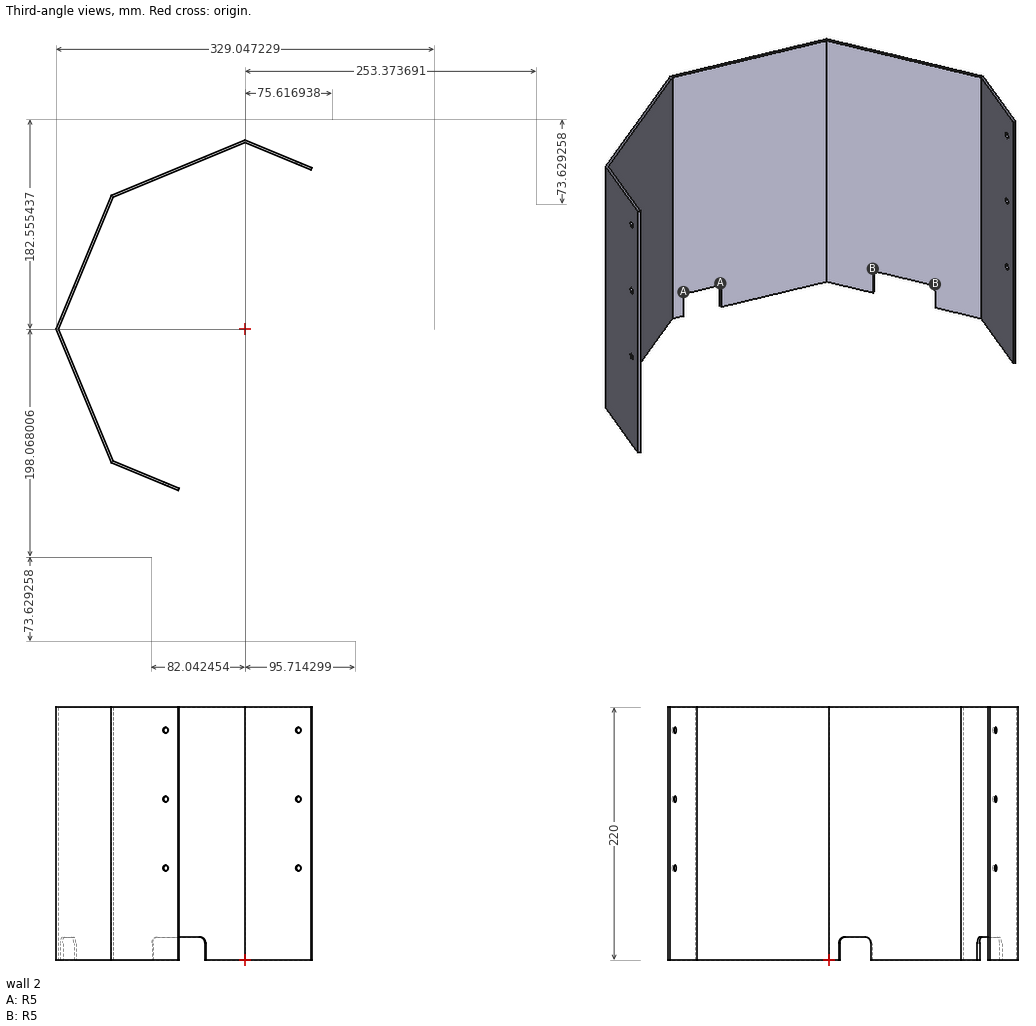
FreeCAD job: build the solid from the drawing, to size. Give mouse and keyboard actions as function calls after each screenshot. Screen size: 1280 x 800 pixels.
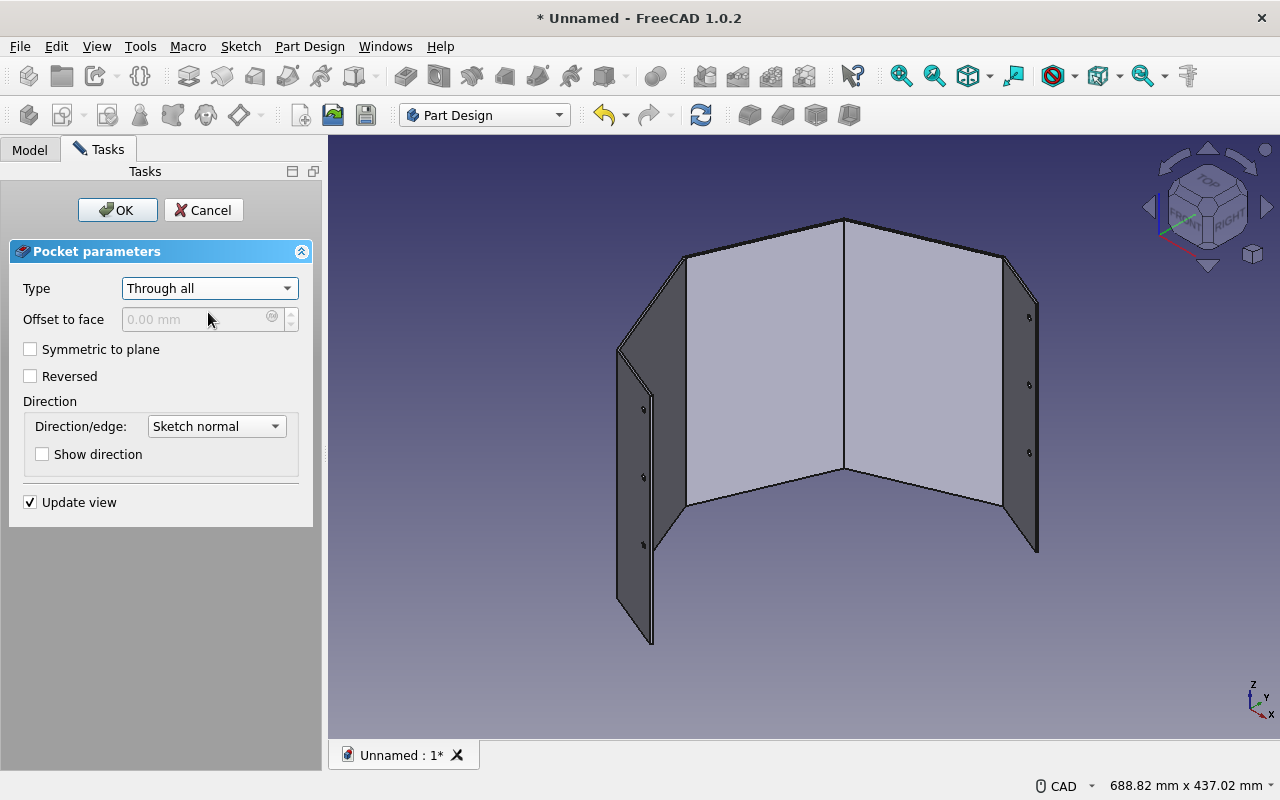
click(118, 210)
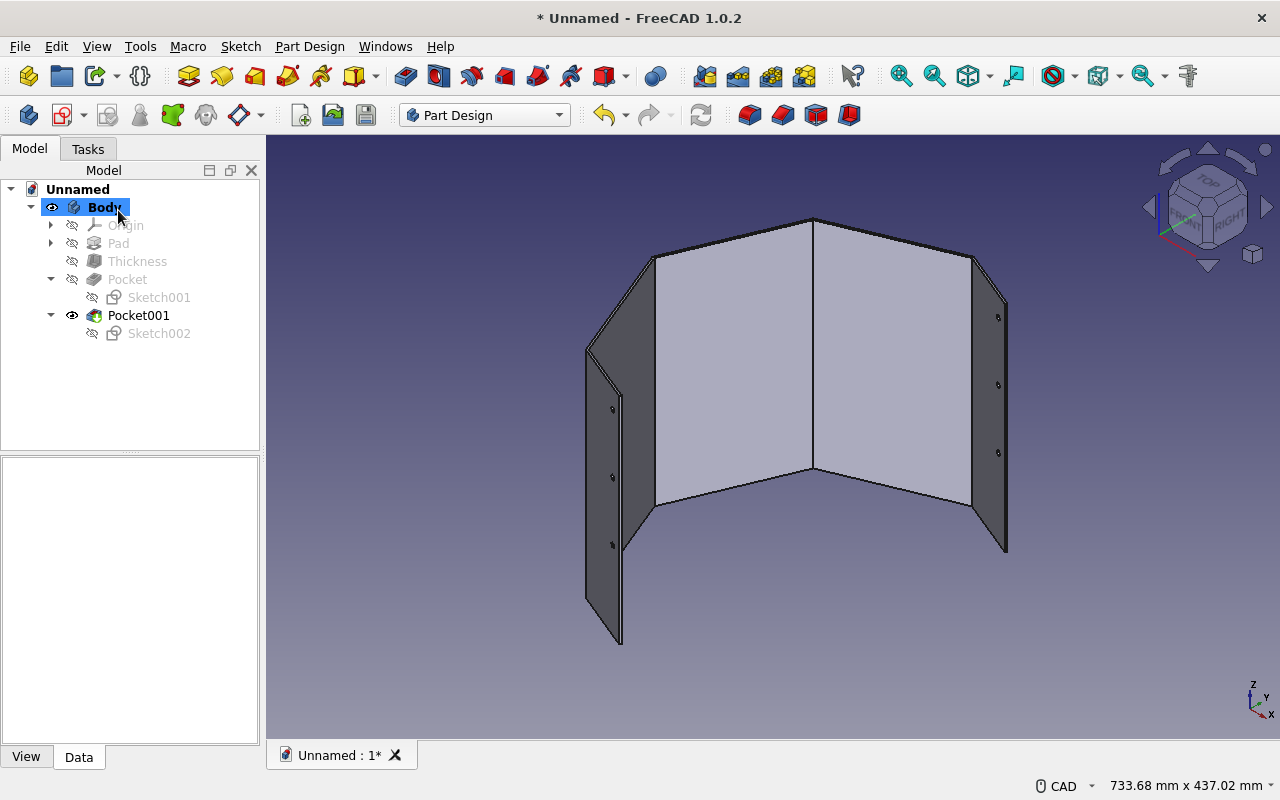
key(6)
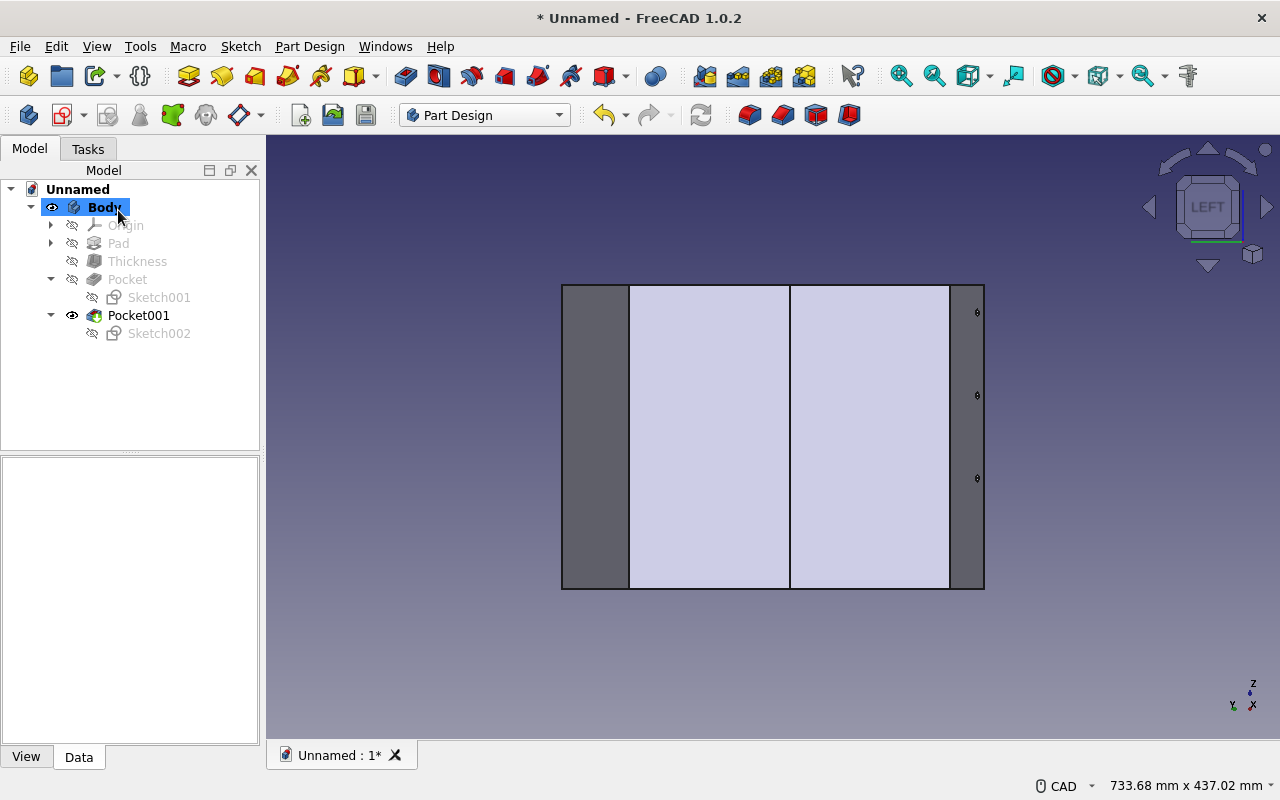
click(709, 393)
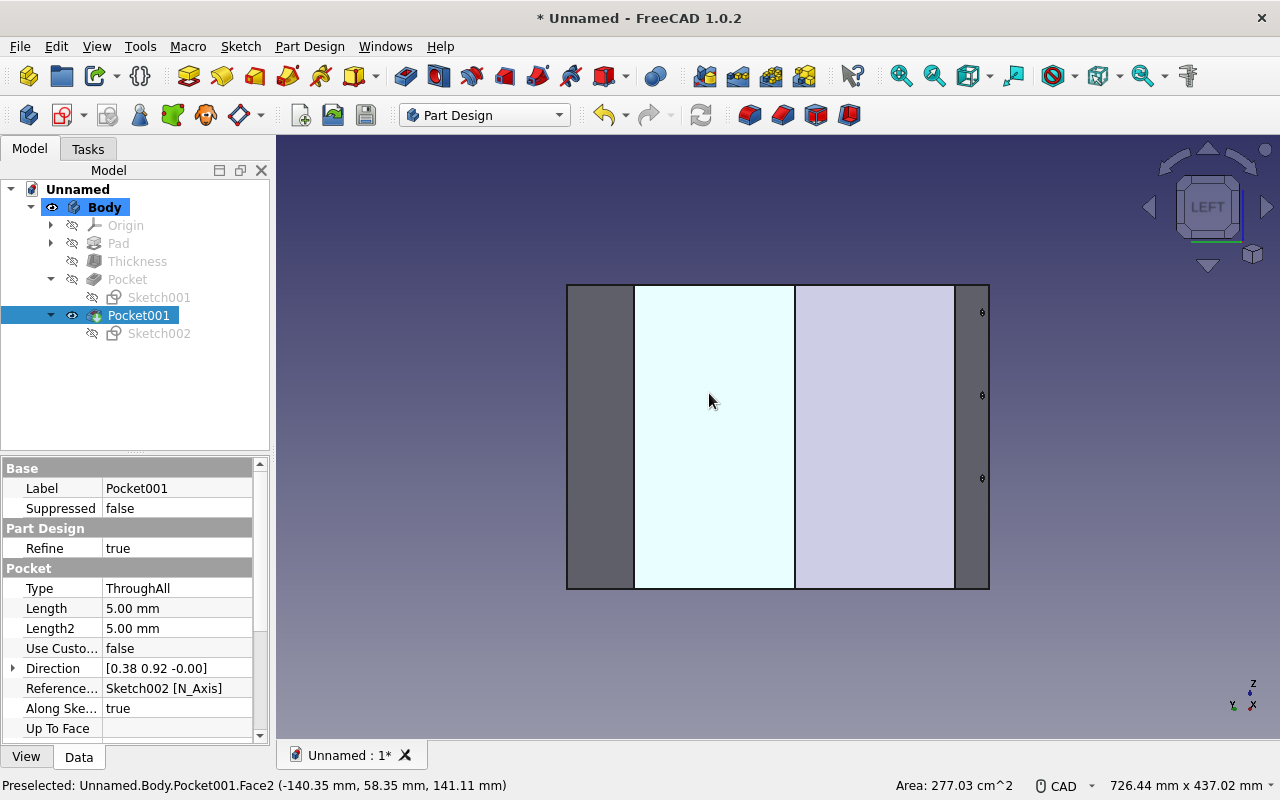
click(62, 116)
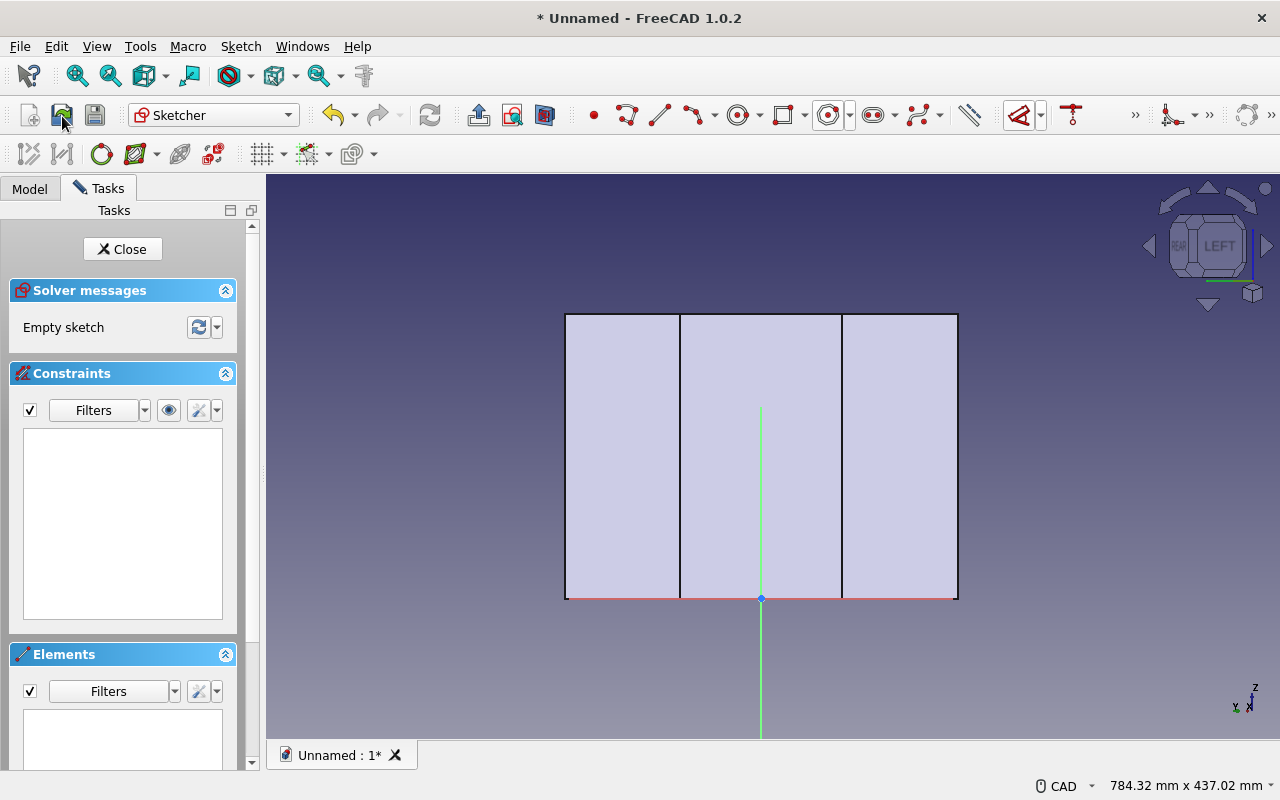
scroll(807, 602, up, 11)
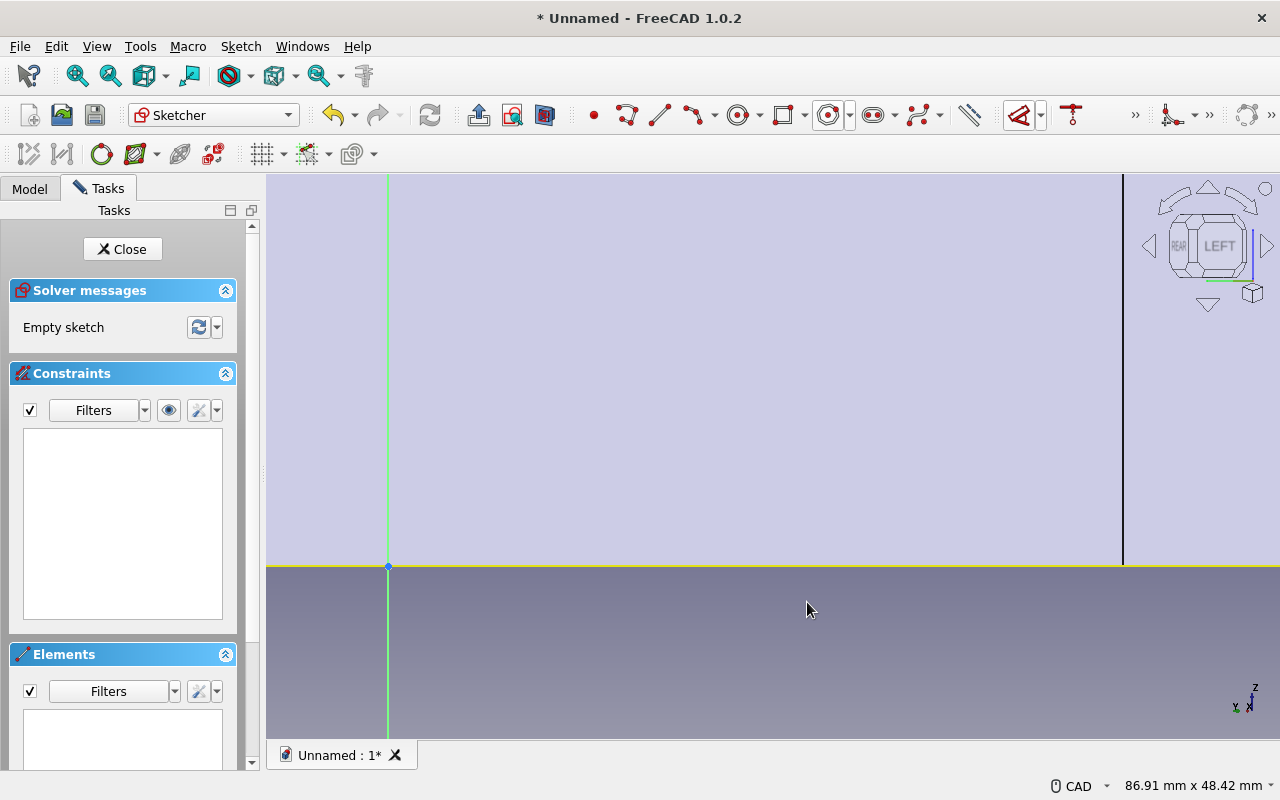
click(782, 116)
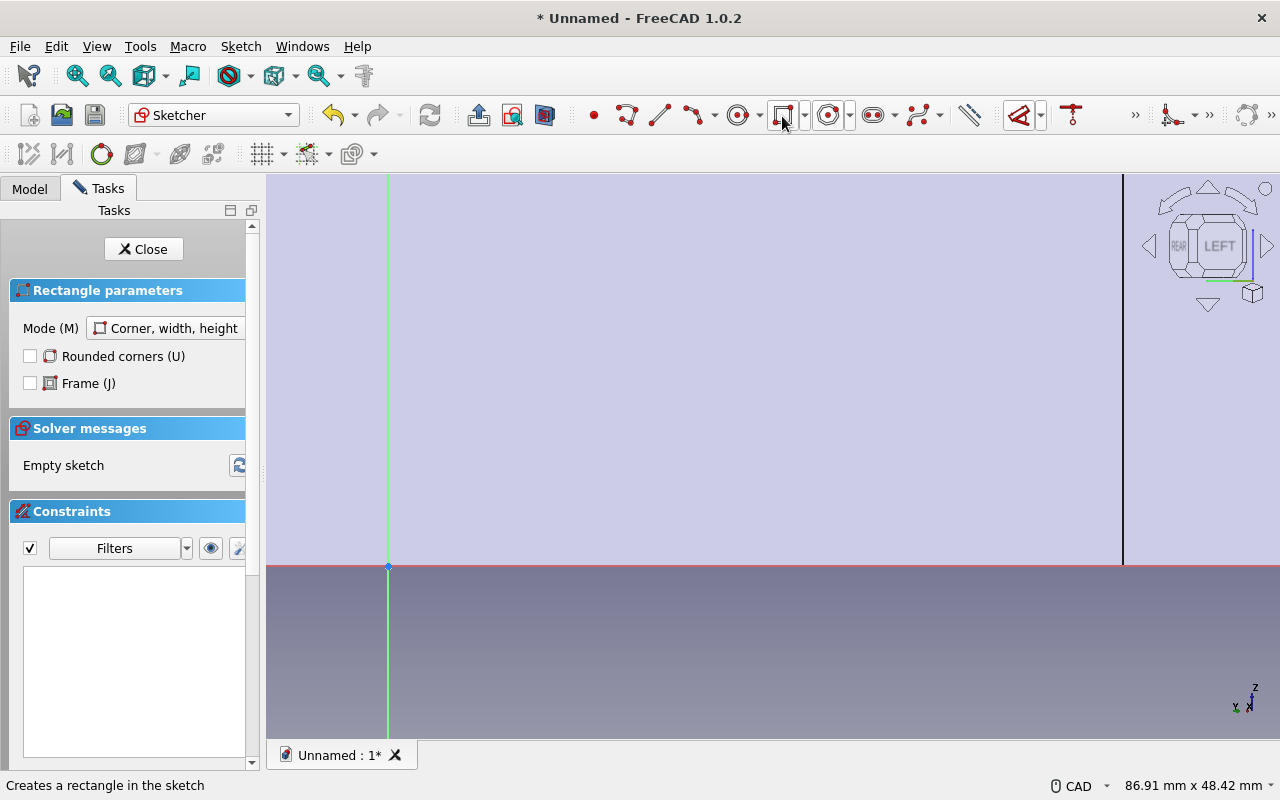
click(656, 333)
click(1006, 566)
key(Escape)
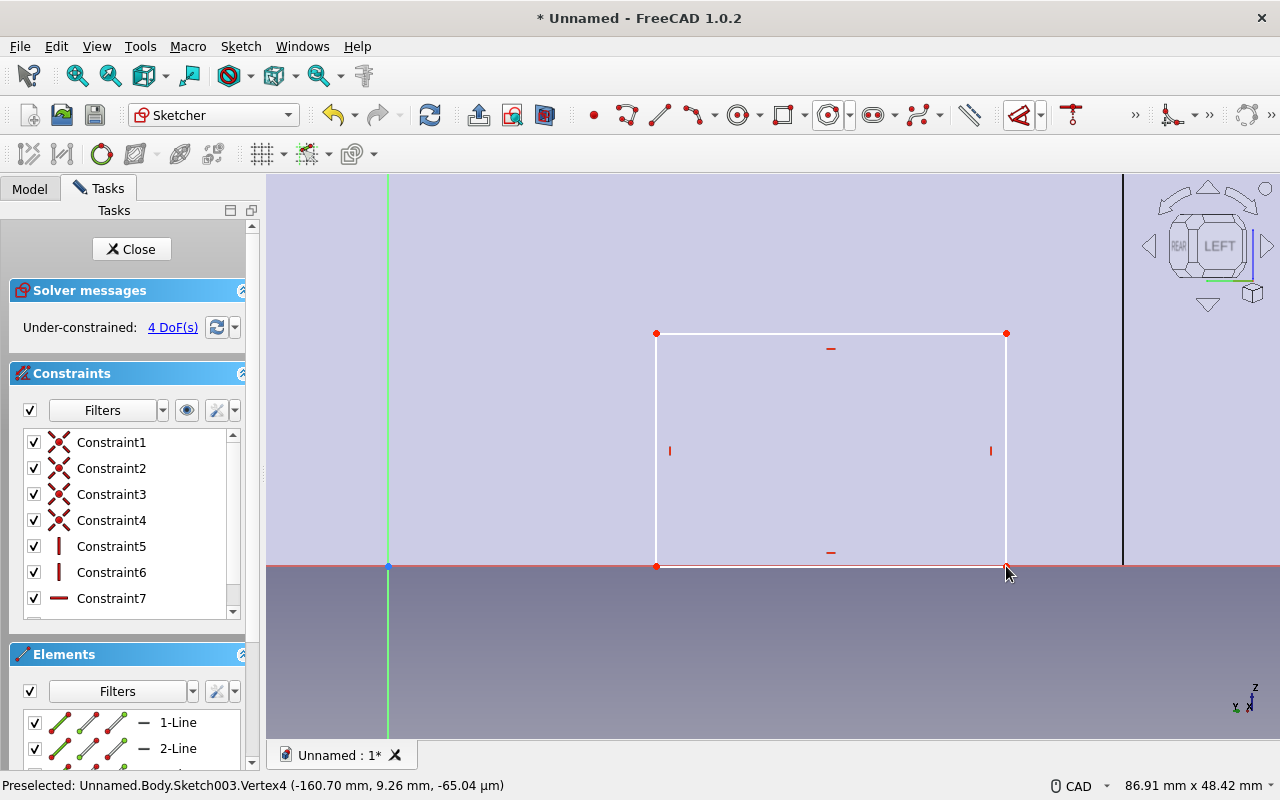
click(656, 567)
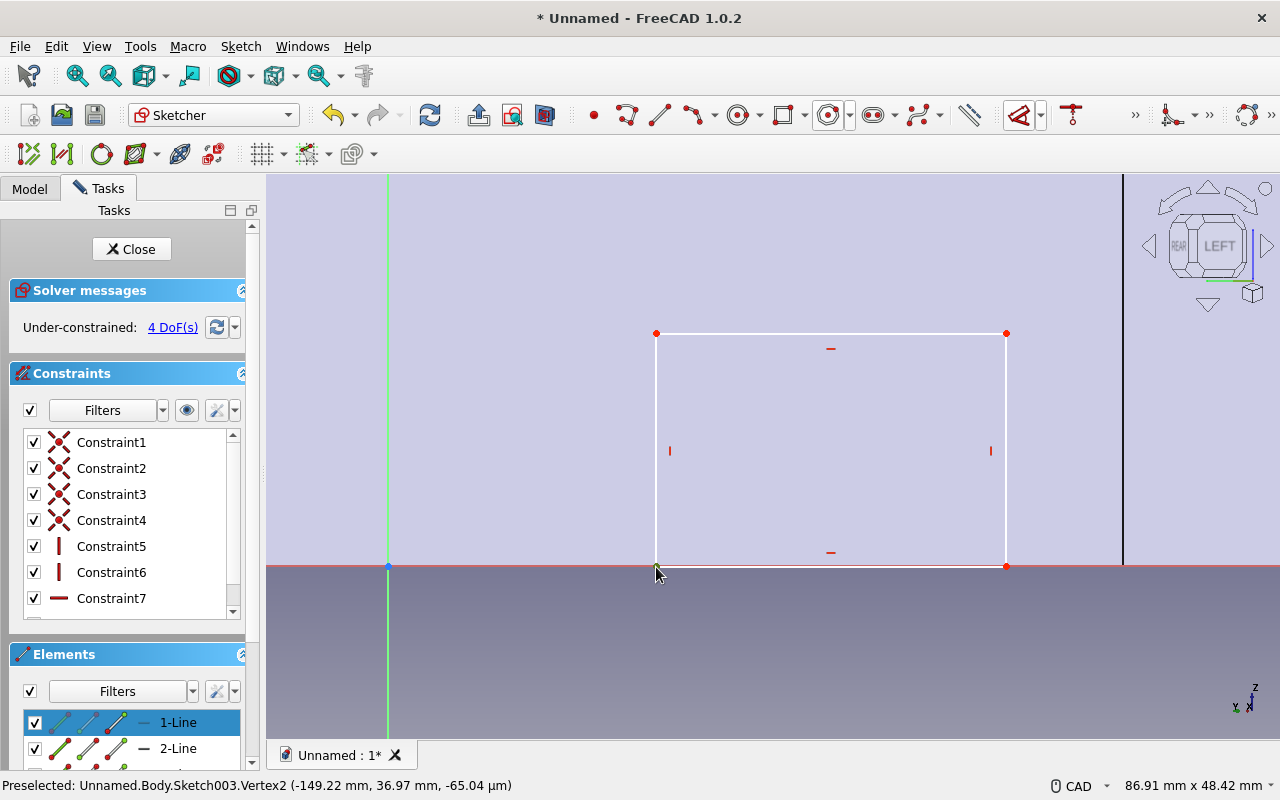
click(353, 566)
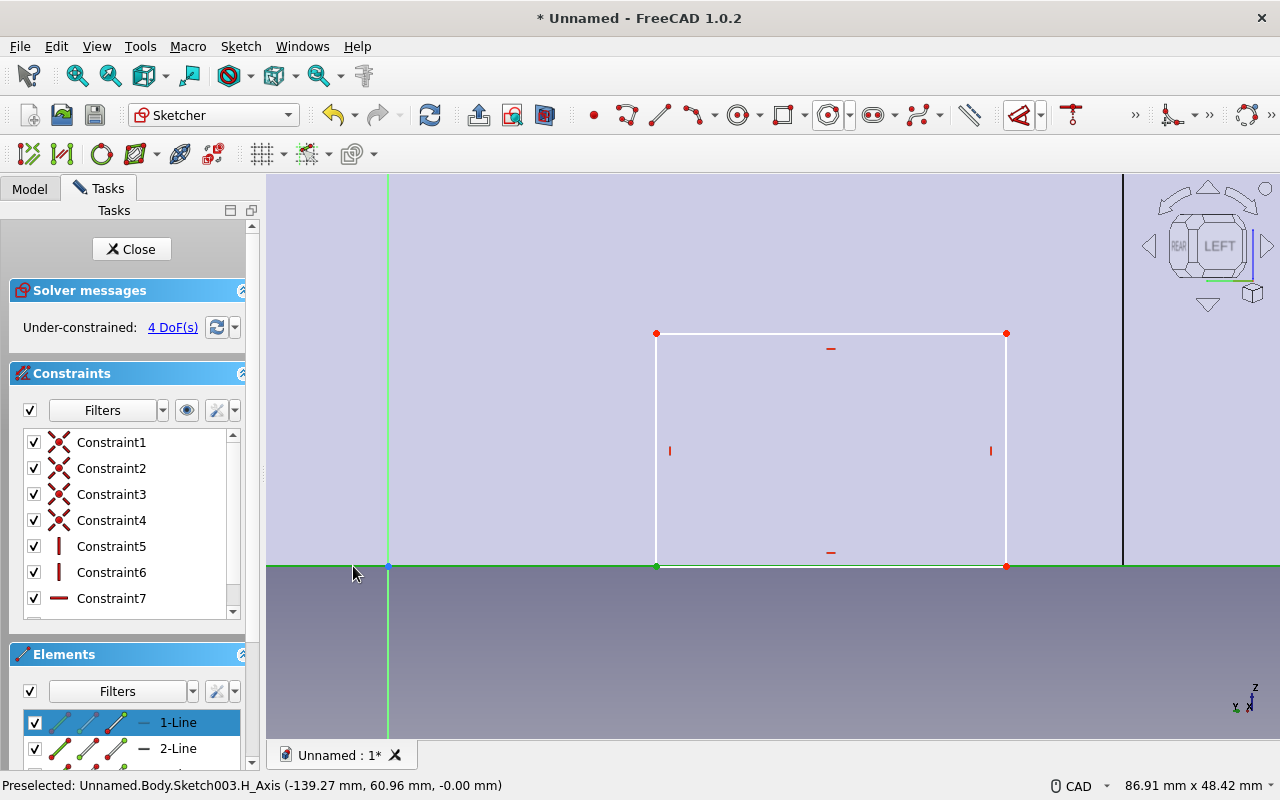
click(1071, 116)